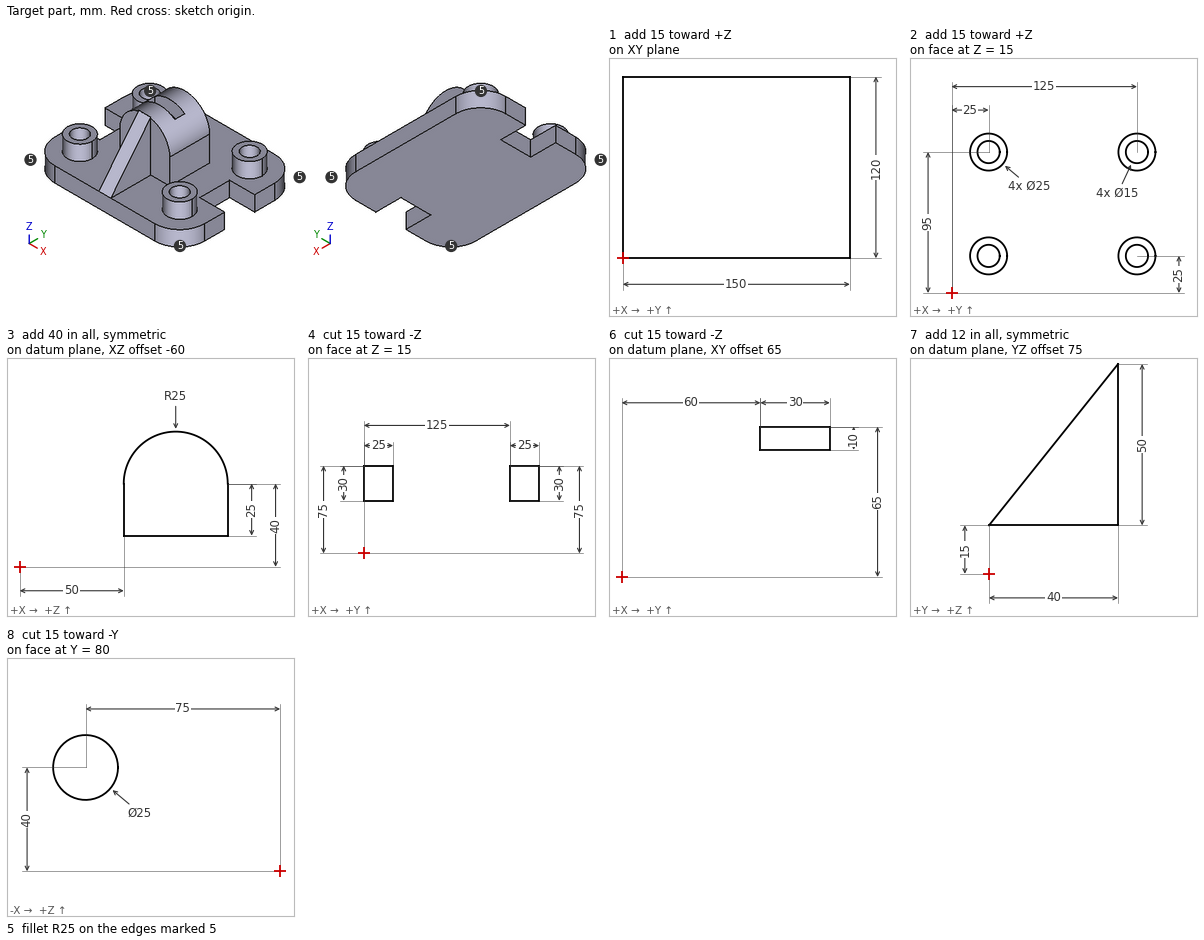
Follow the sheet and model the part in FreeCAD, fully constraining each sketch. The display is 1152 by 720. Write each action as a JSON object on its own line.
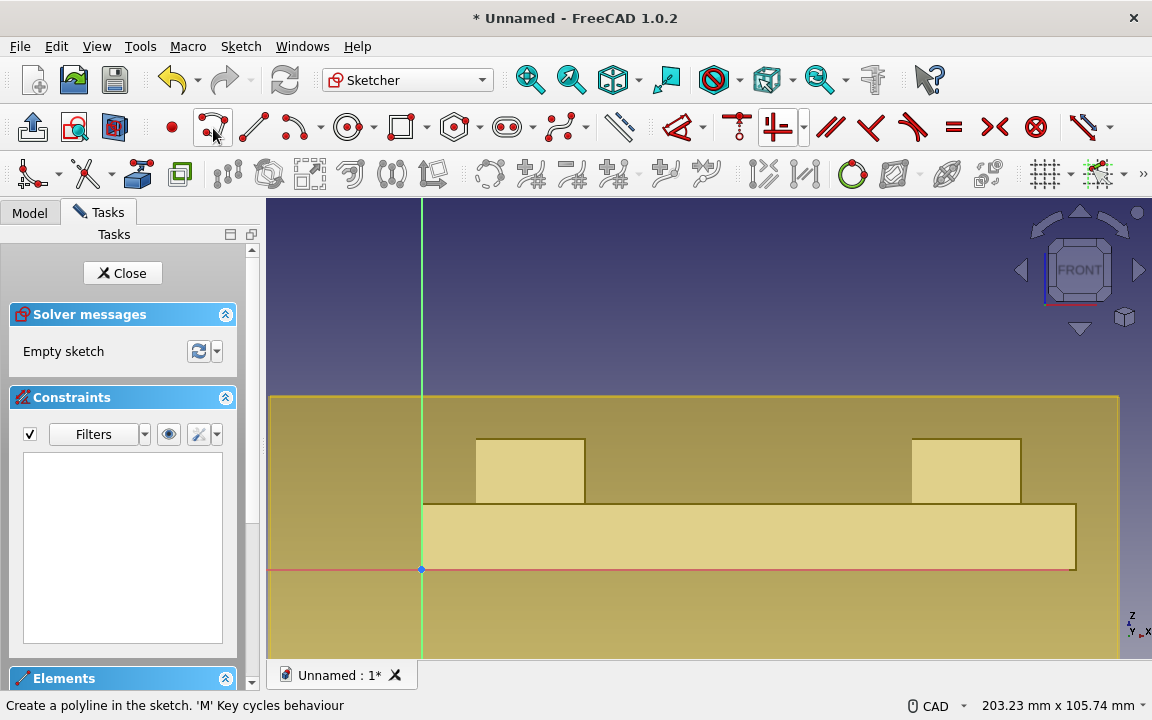
{"action": "left_click", "coordinate": [858, 395]}
{"action": "left_click", "coordinate": [858, 504]}
{"action": "left_click", "coordinate": [640, 504]}
{"action": "left_click", "coordinate": [640, 395]}
{"action": "right_click", "coordinate": [640, 395]}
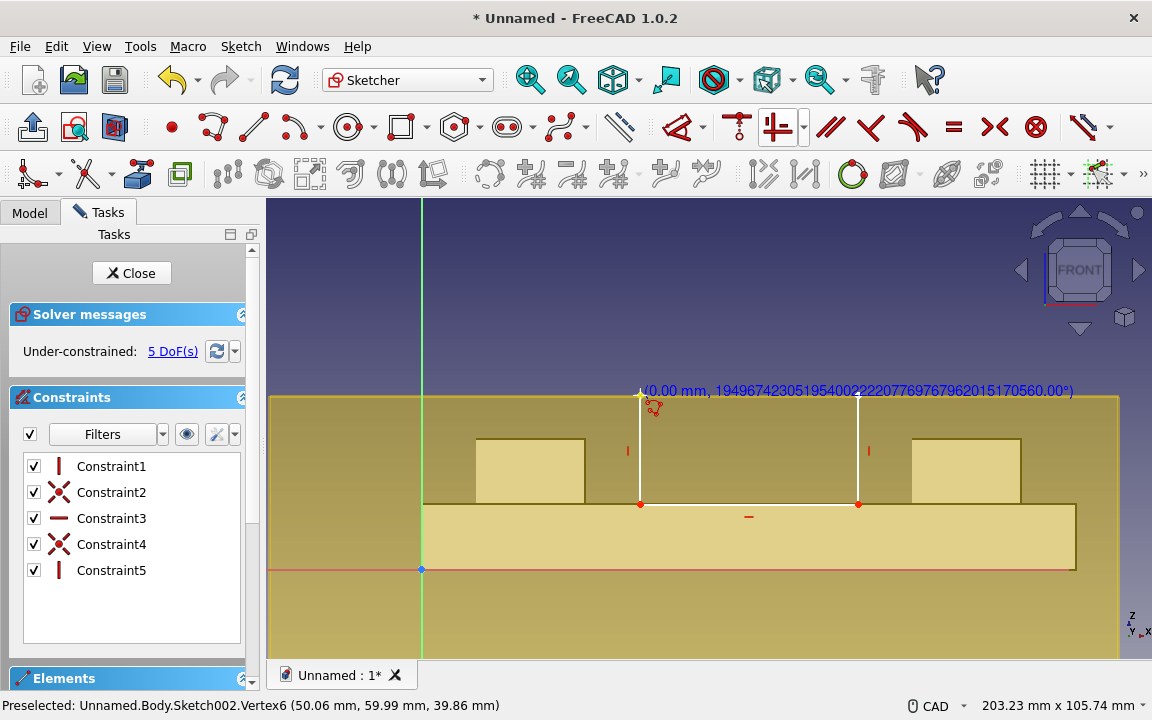
{"action": "key", "text": "g 3 a"}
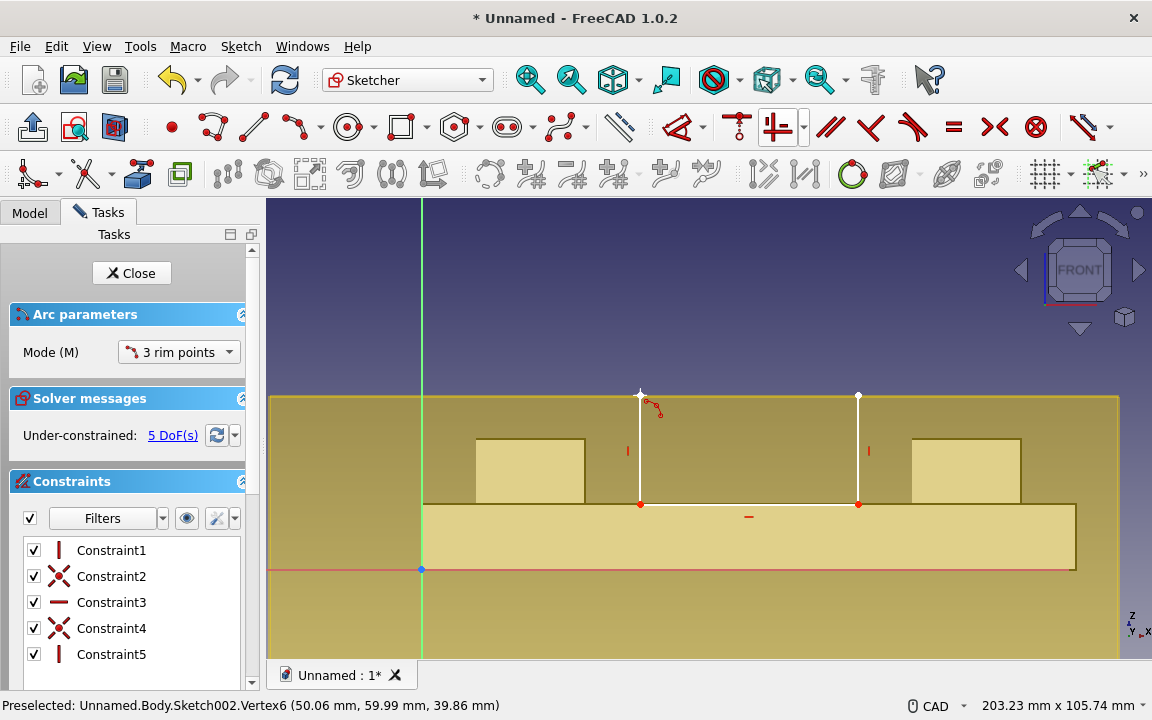
{"action": "left_click", "coordinate": [640, 396]}
{"action": "left_click", "coordinate": [858, 396]}
{"action": "left_click", "coordinate": [749, 286]}
{"action": "key", "text": "Escape"}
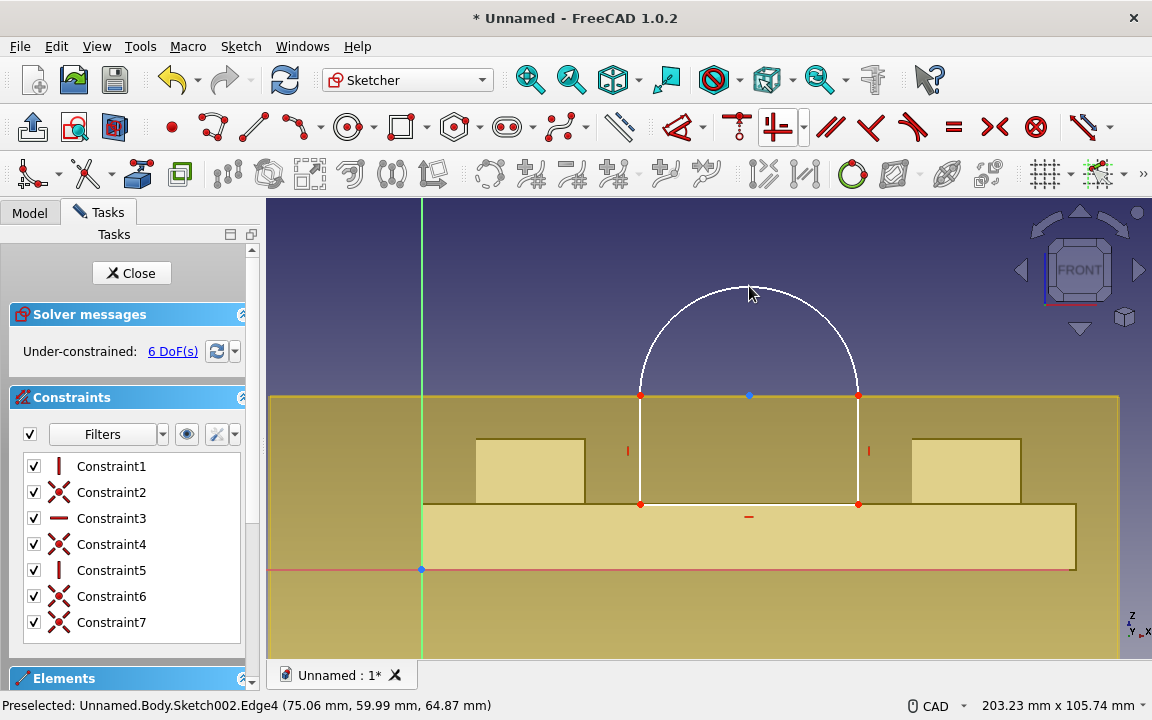
{"action": "left_click", "coordinate": [858, 429]}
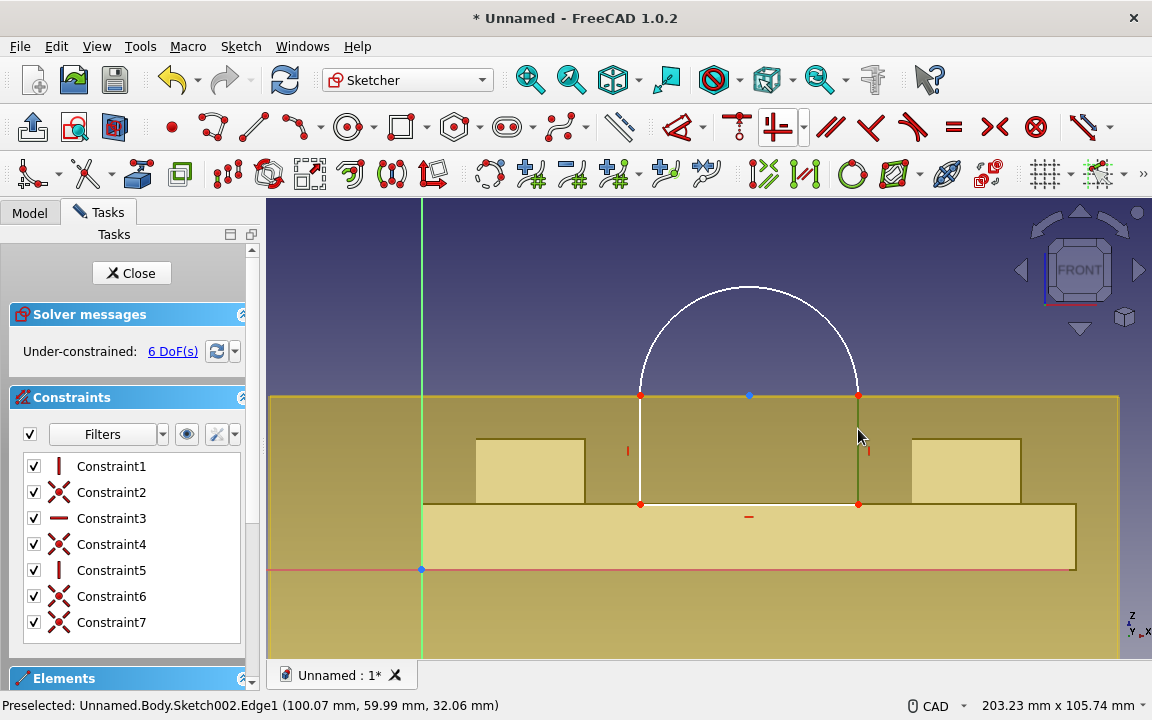
{"action": "left_click", "coordinate": [813, 308]}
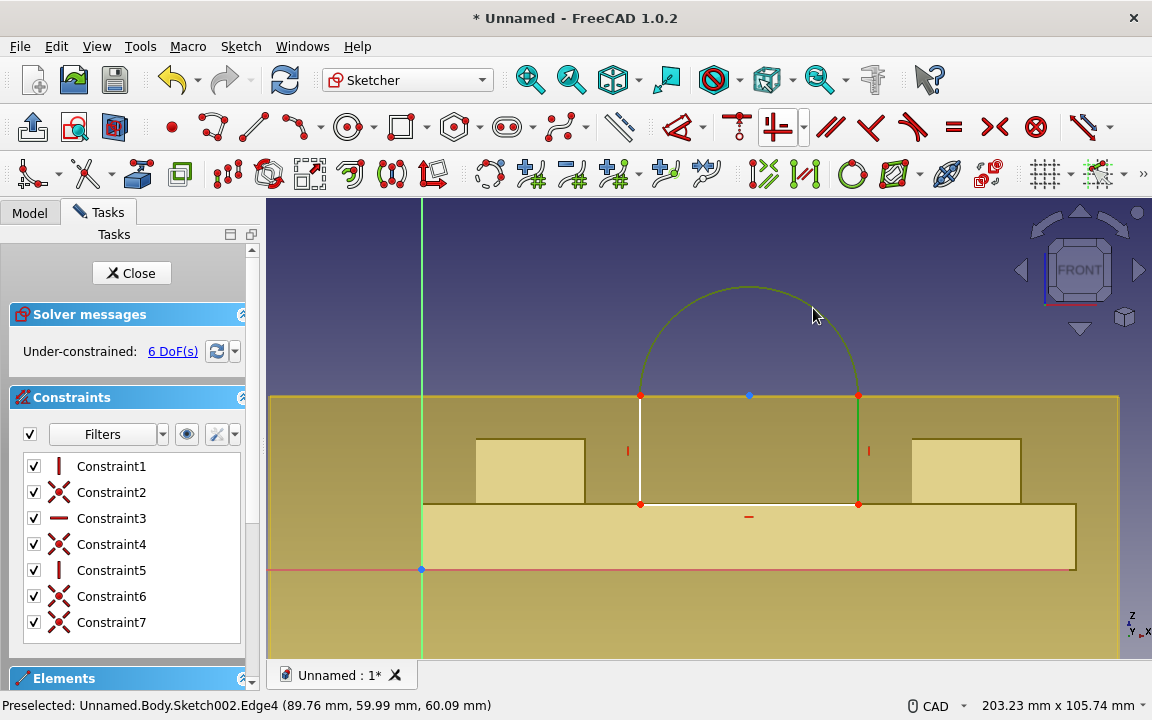
{"action": "left_click", "coordinate": [913, 128]}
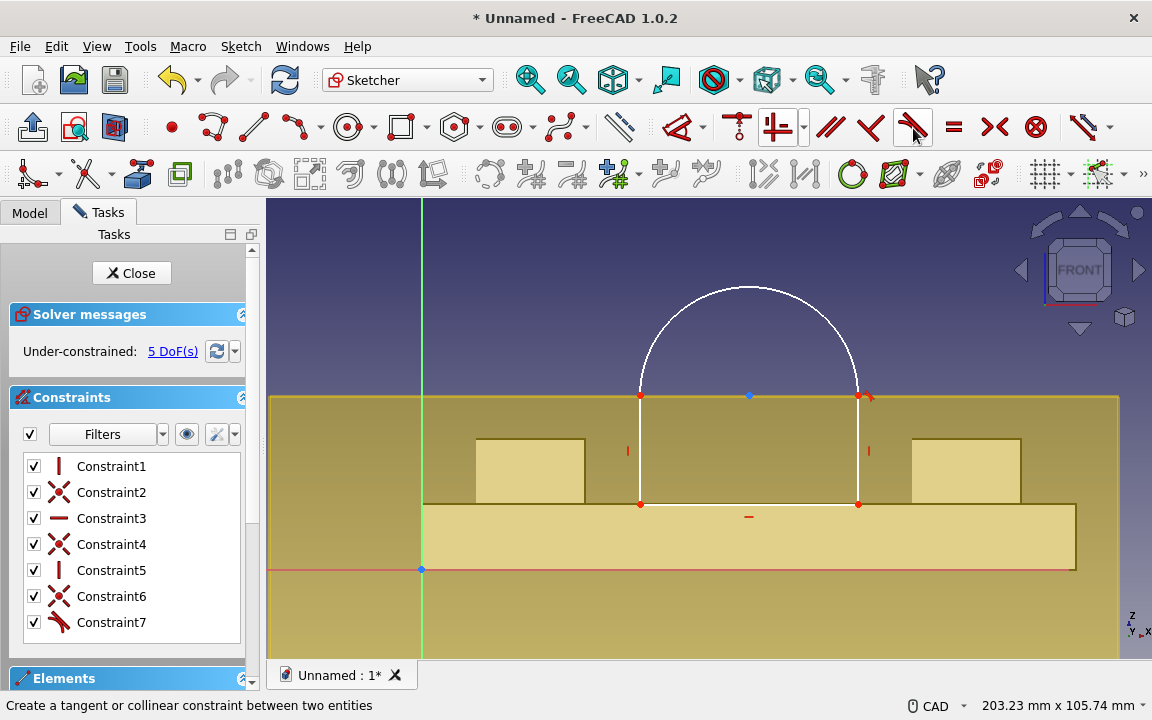
{"action": "left_click", "coordinate": [640, 472]}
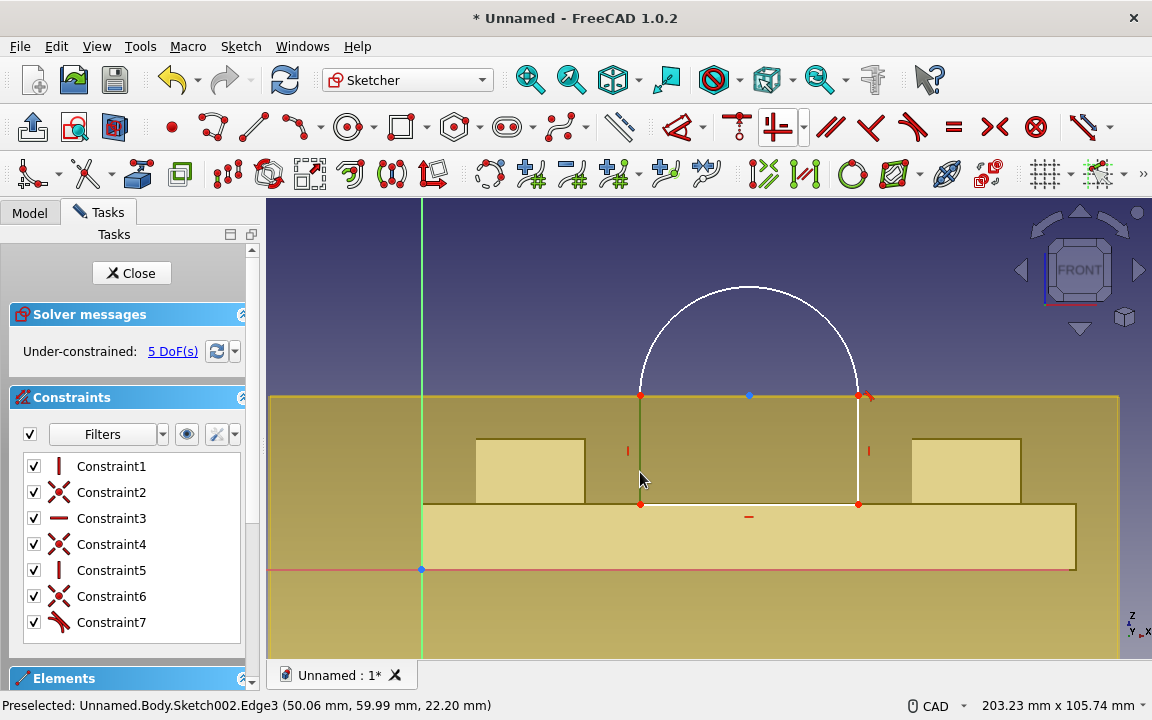
{"action": "left_click", "coordinate": [813, 308]}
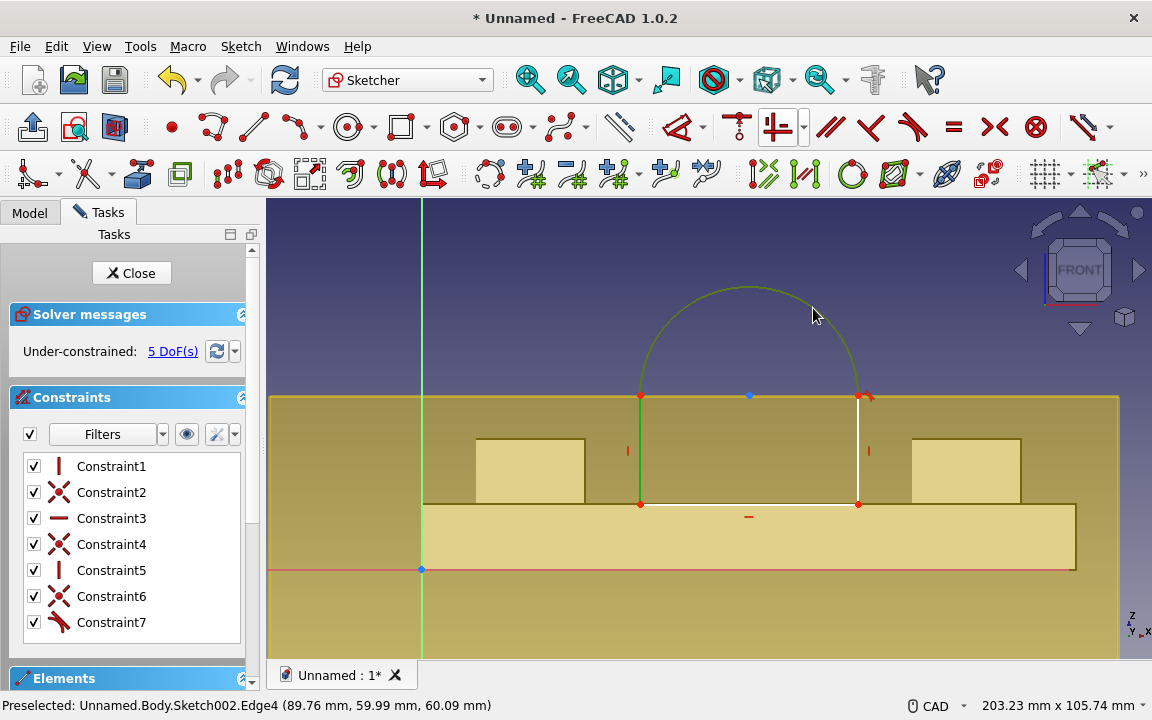
{"action": "left_click", "coordinate": [913, 128]}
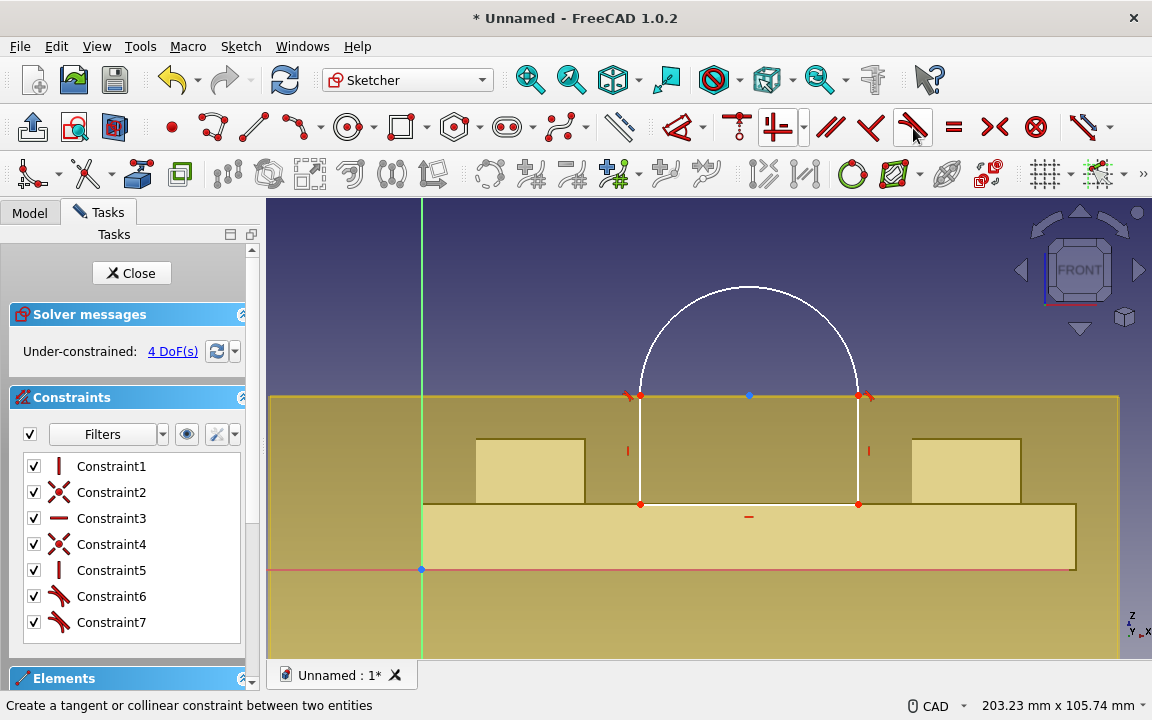
{"action": "key", "text": "d"}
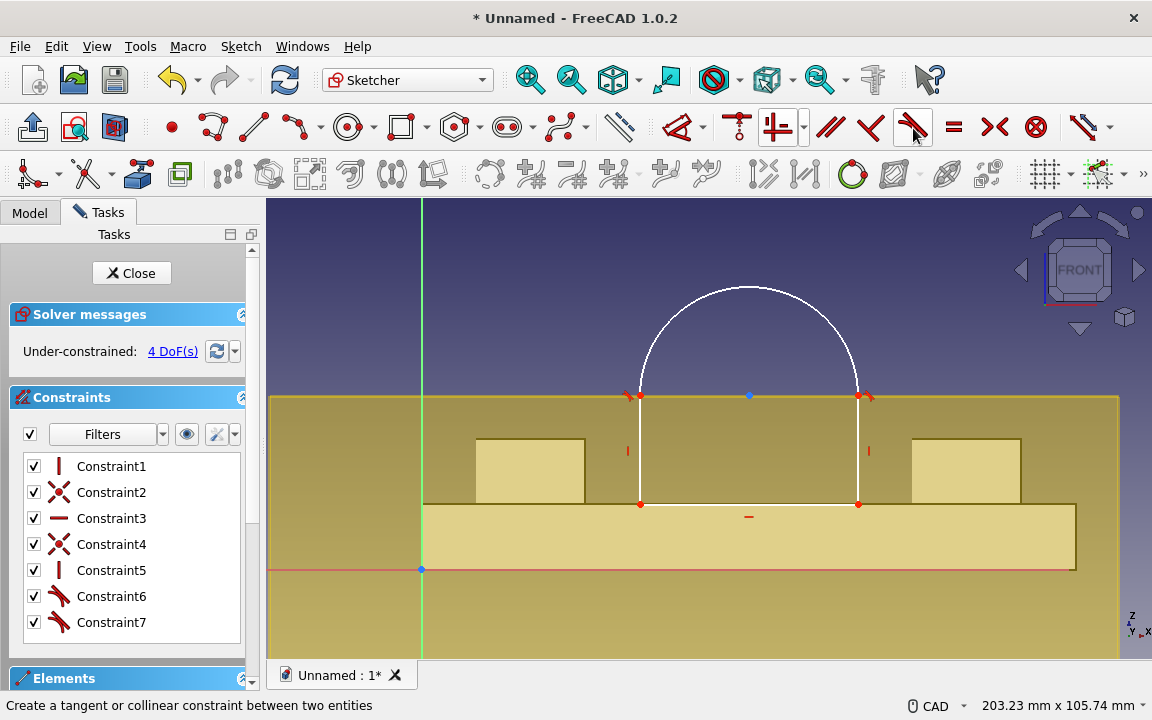
{"action": "left_click", "coordinate": [813, 308]}
{"action": "left_click", "coordinate": [832, 282]}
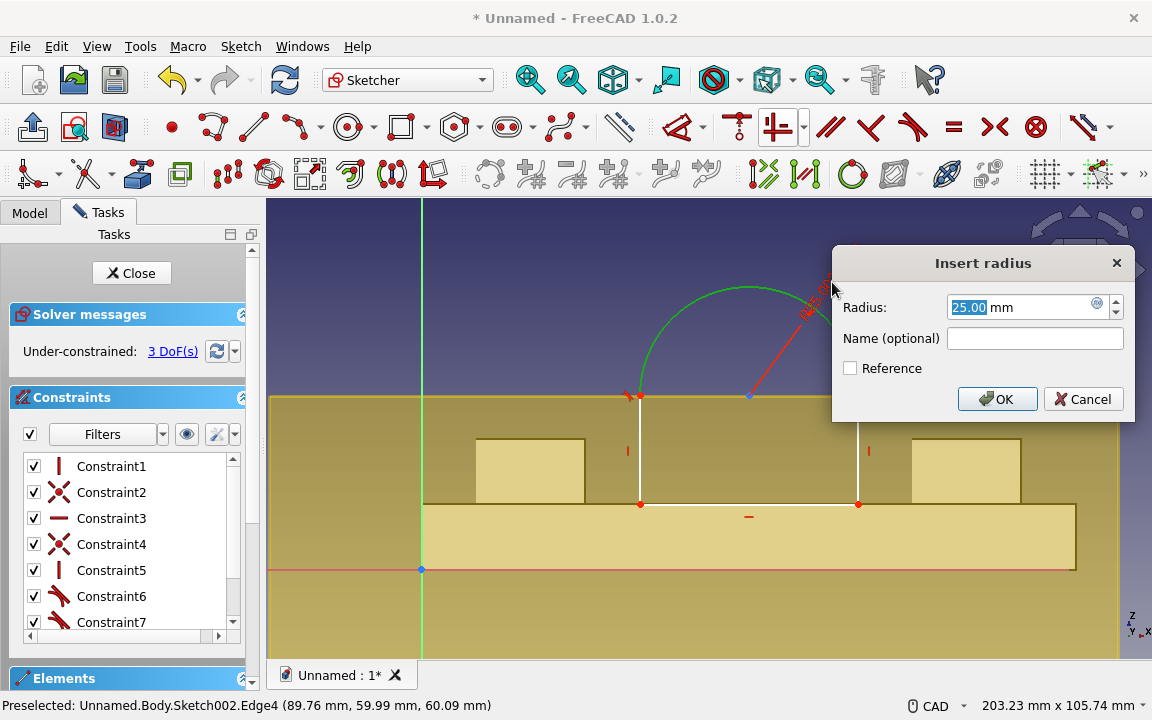
{"action": "type", "text": "25"}
{"action": "key", "text": "Return"}